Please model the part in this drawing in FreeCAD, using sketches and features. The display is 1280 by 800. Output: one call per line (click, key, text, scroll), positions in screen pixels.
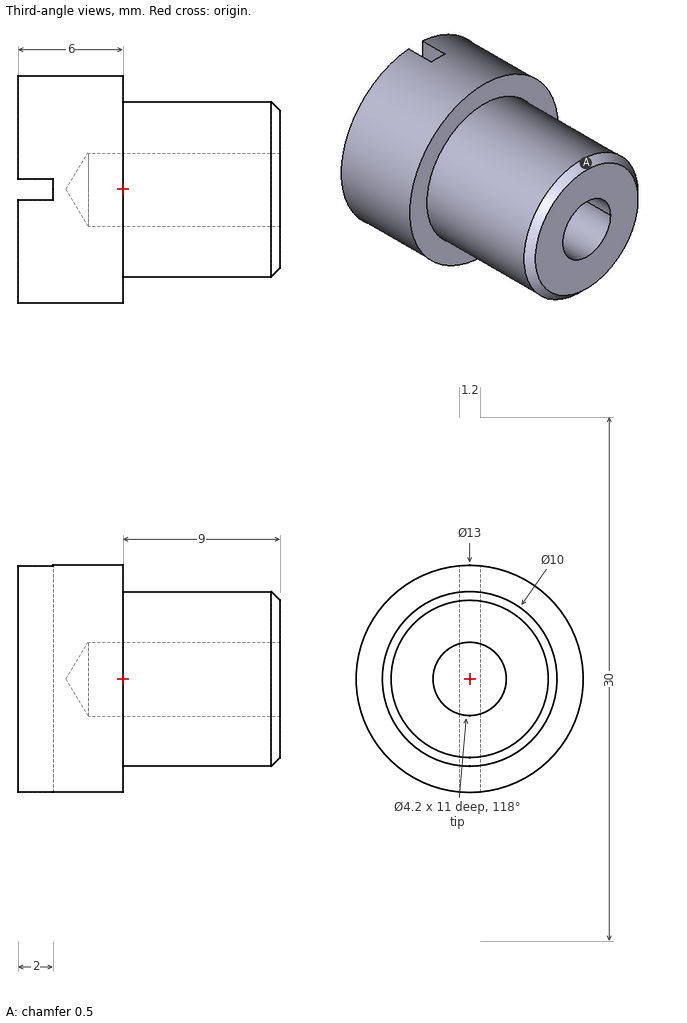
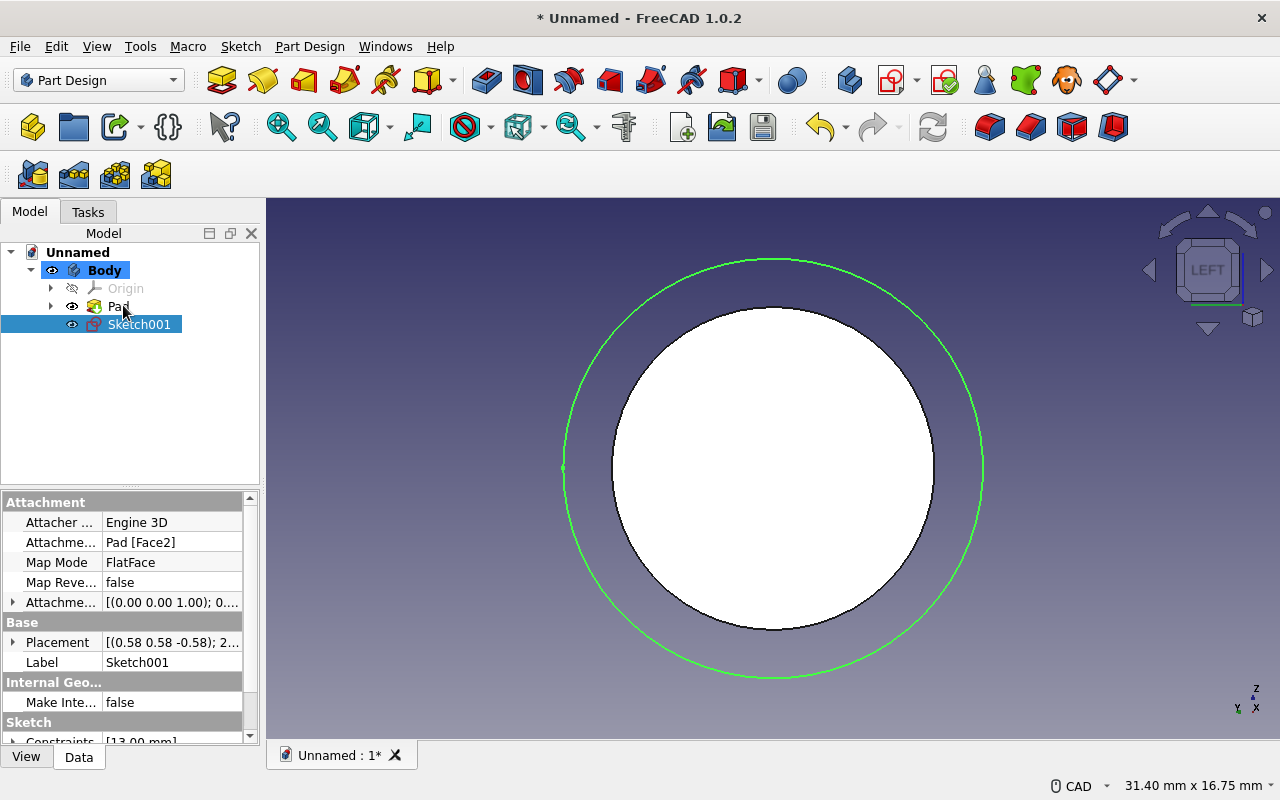
click(222, 80)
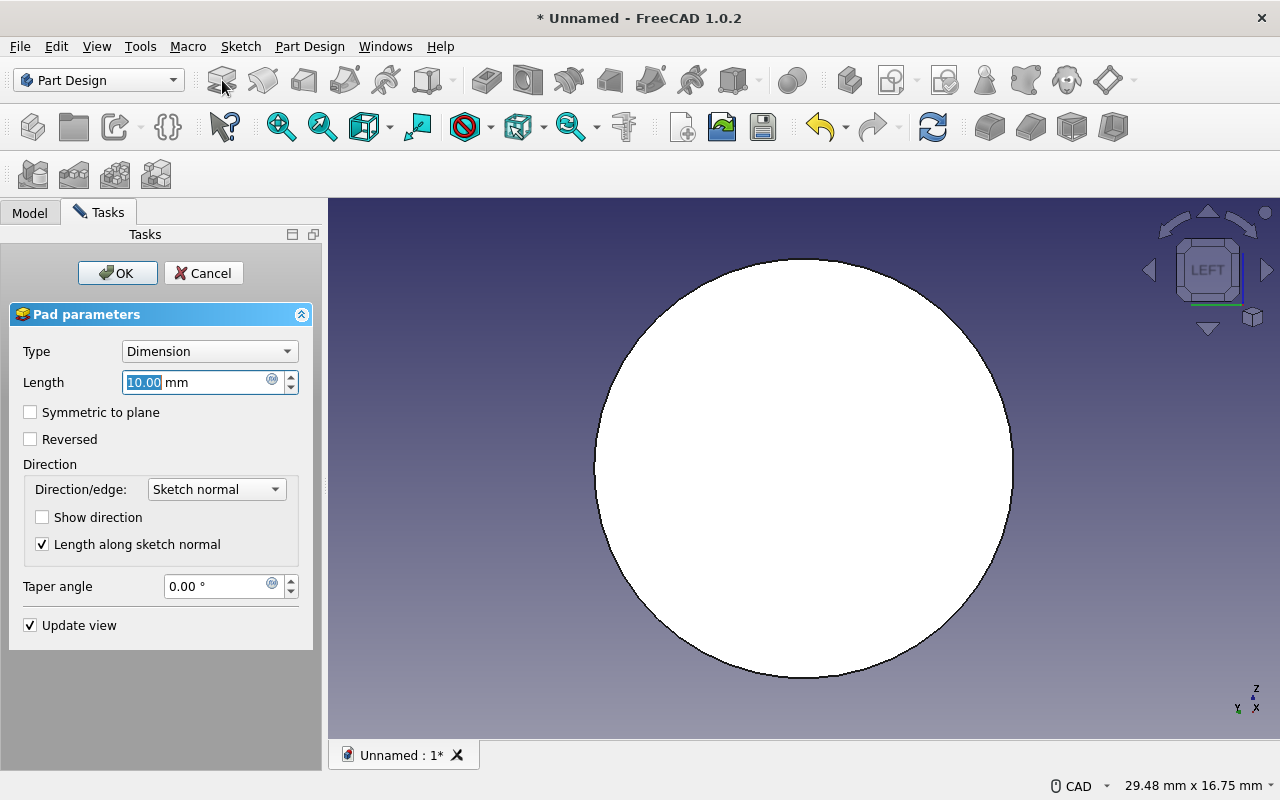
text(6)
key(Tab)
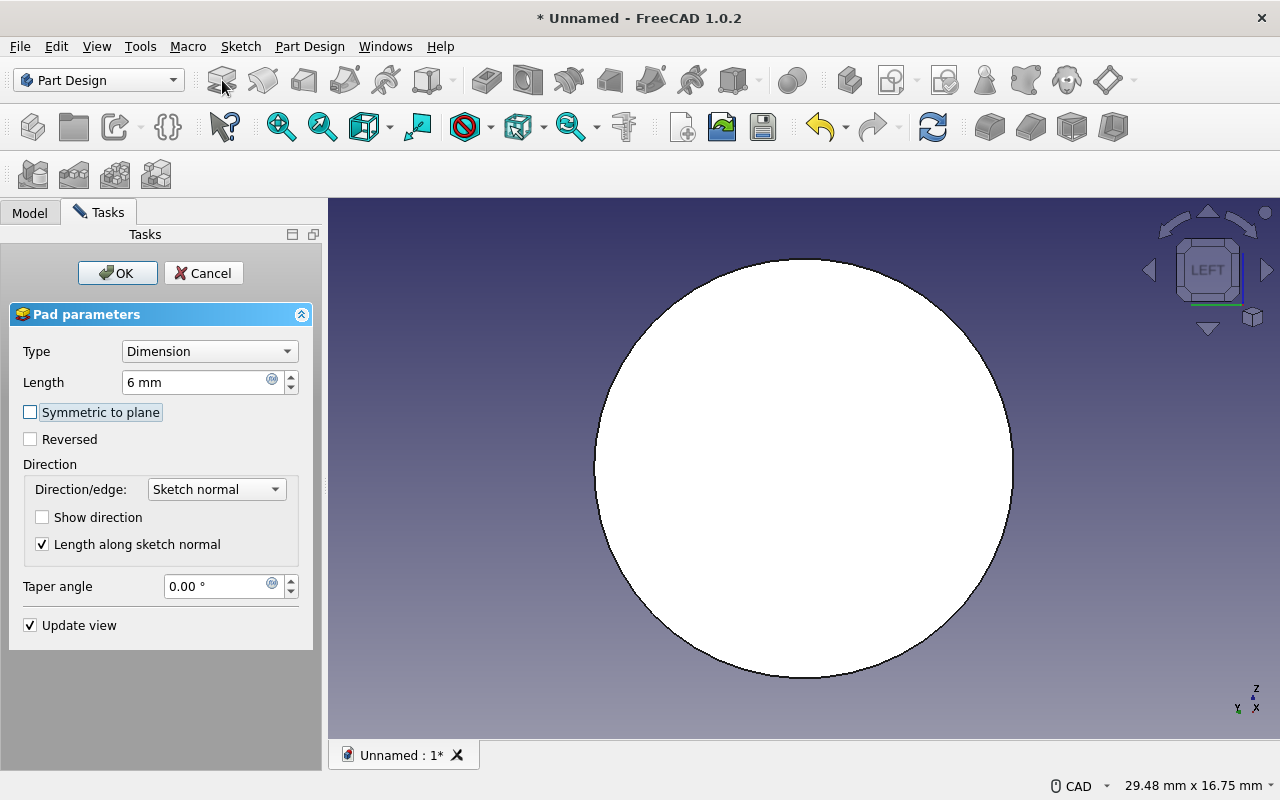
click(118, 273)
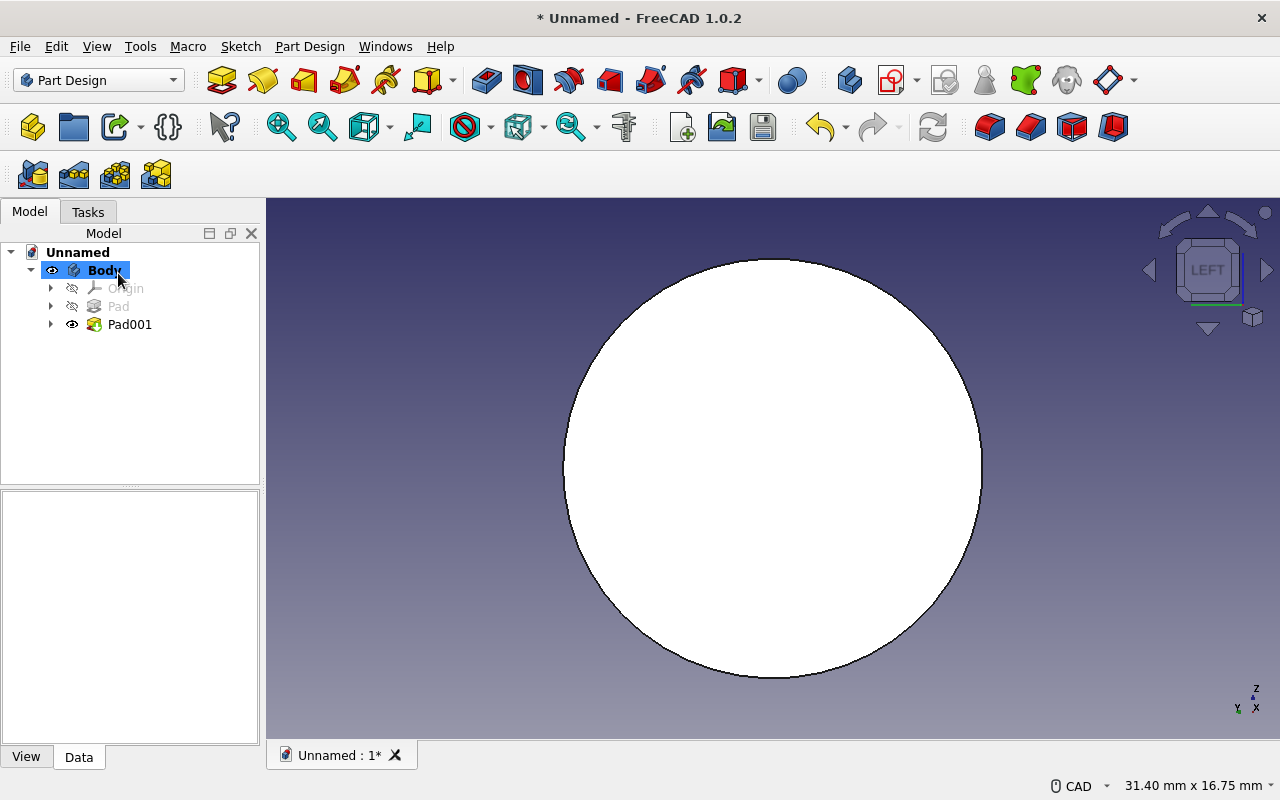
click(773, 467)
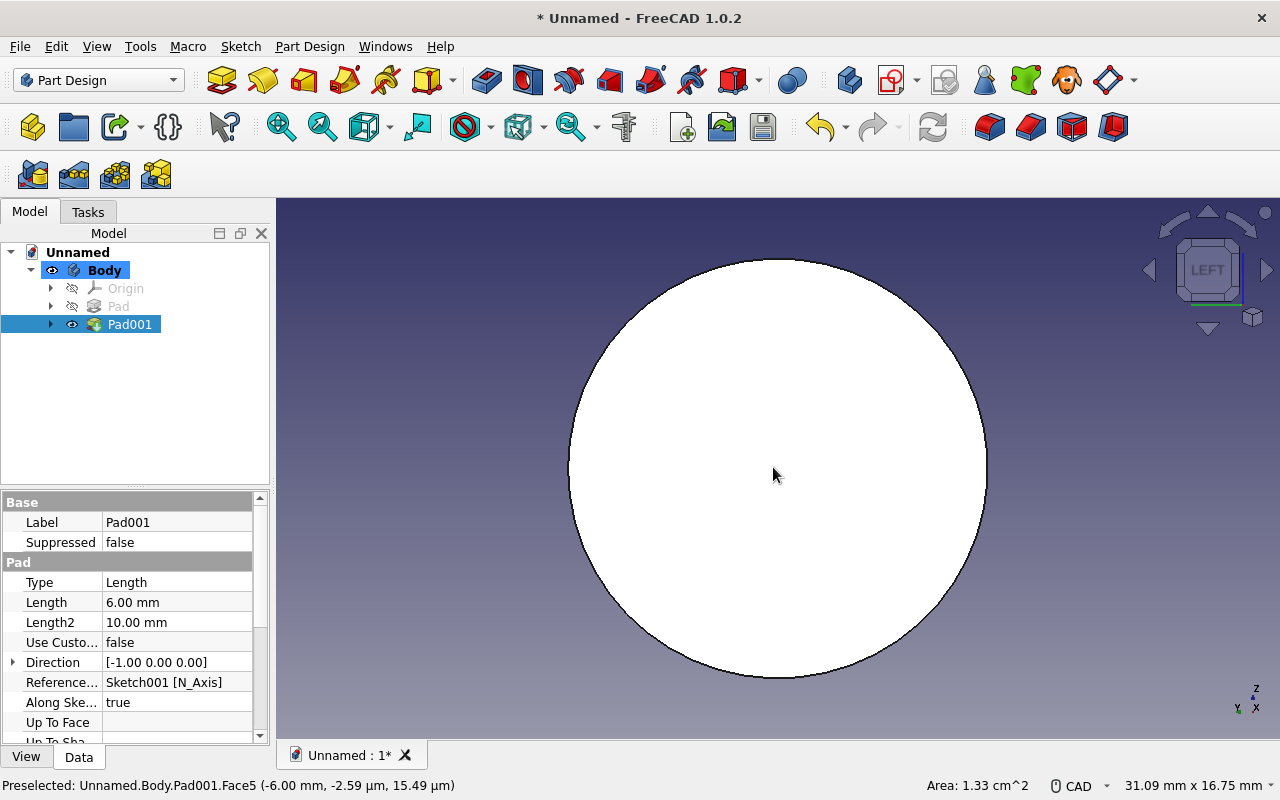
click(890, 80)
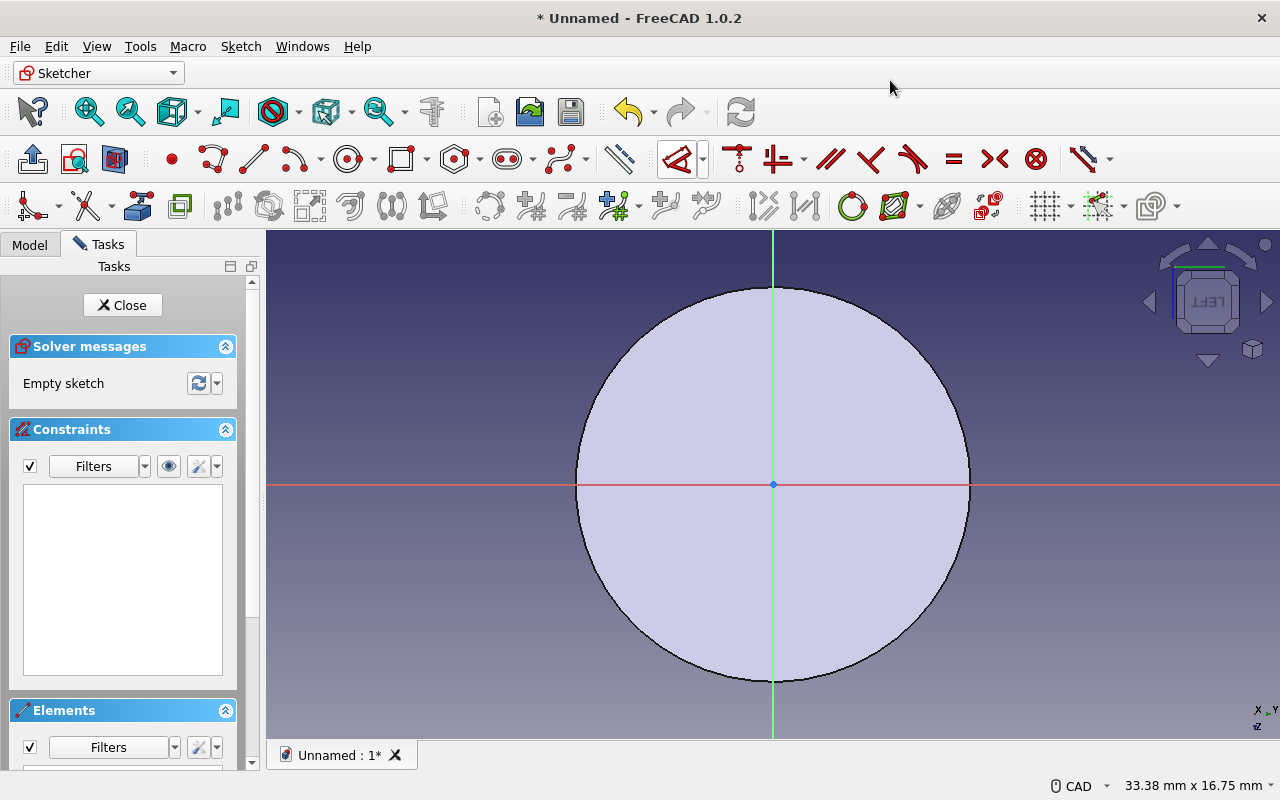
scroll(665, 485, down, 5)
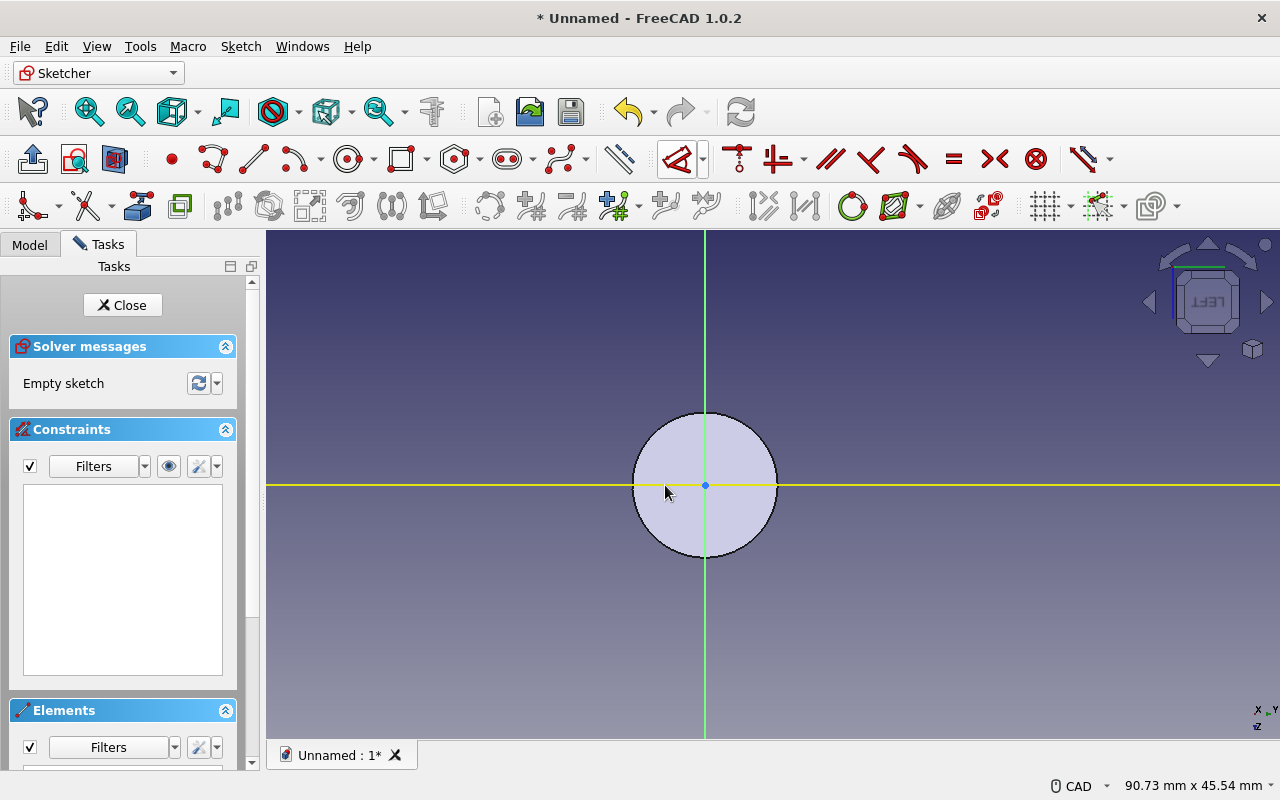
key(g)
key(v)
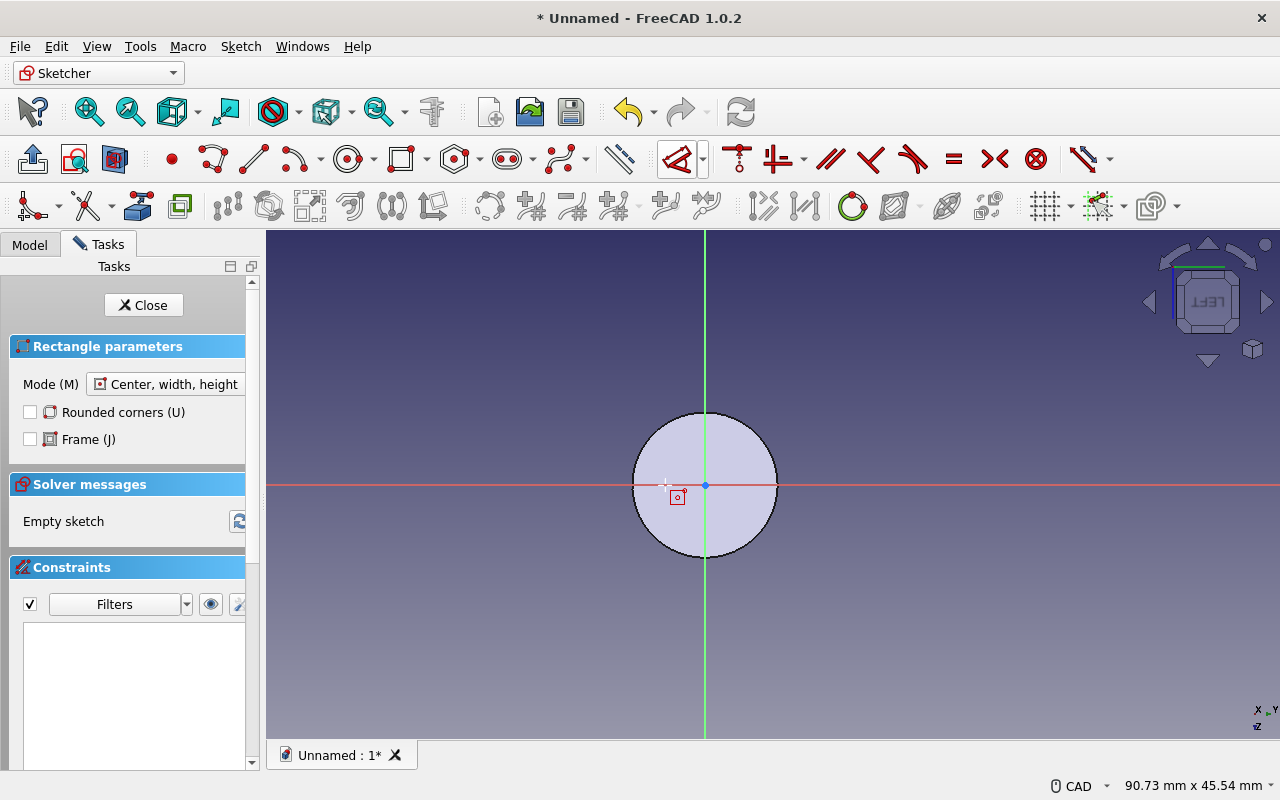
scroll(705, 485, up, 5)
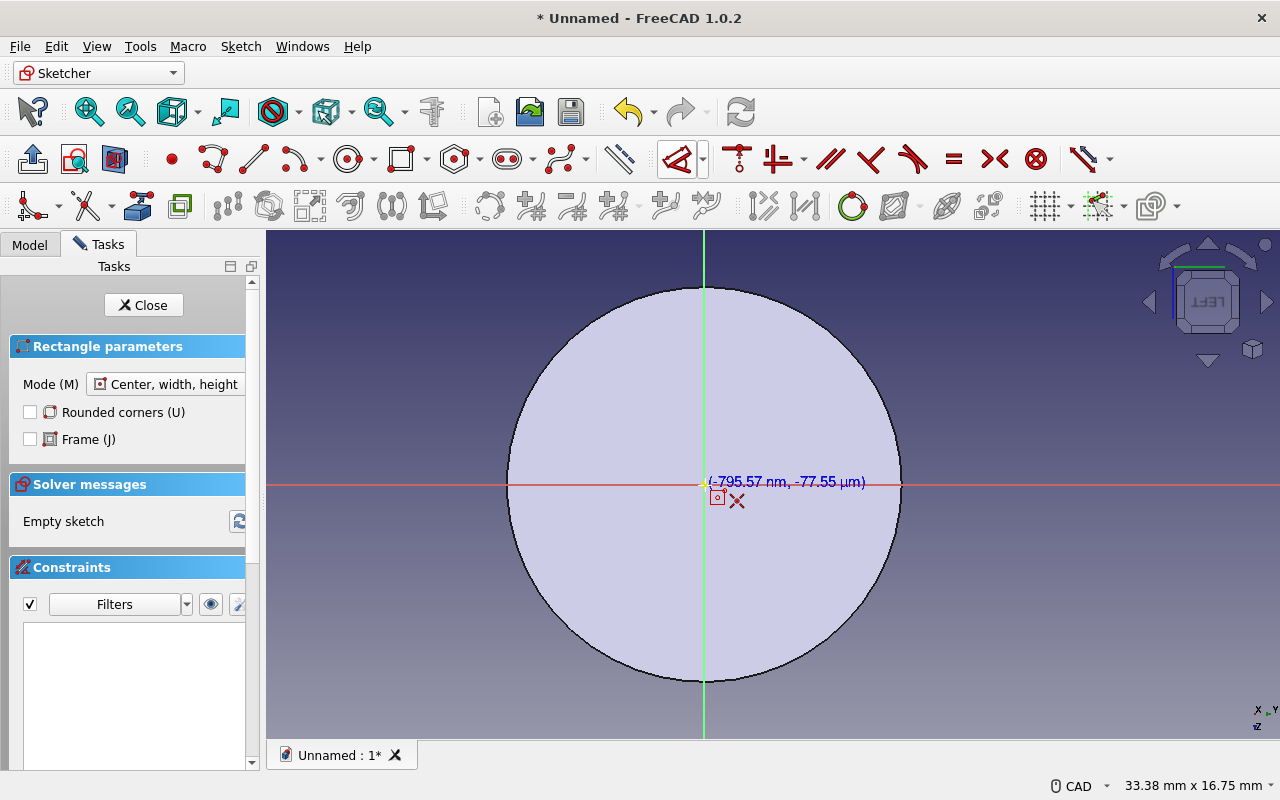
click(704, 484)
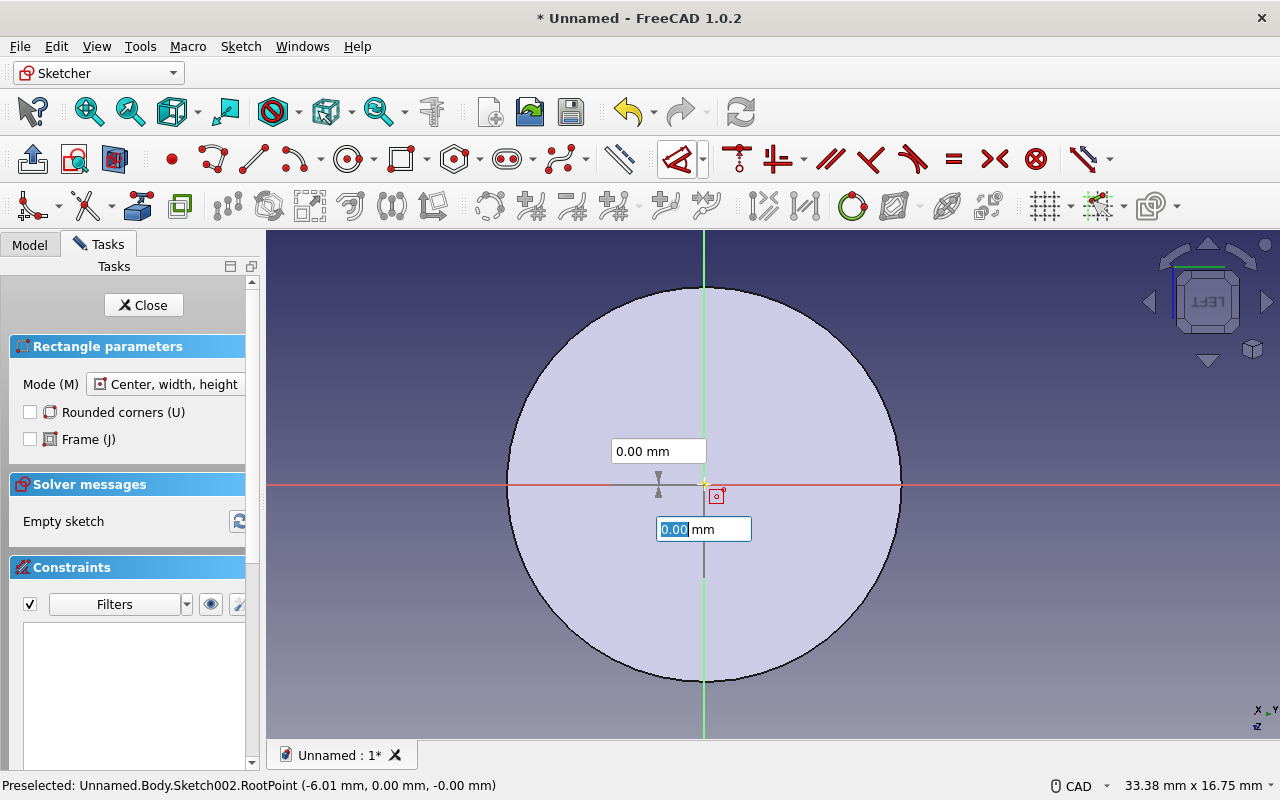
scroll(705, 485, down, 5)